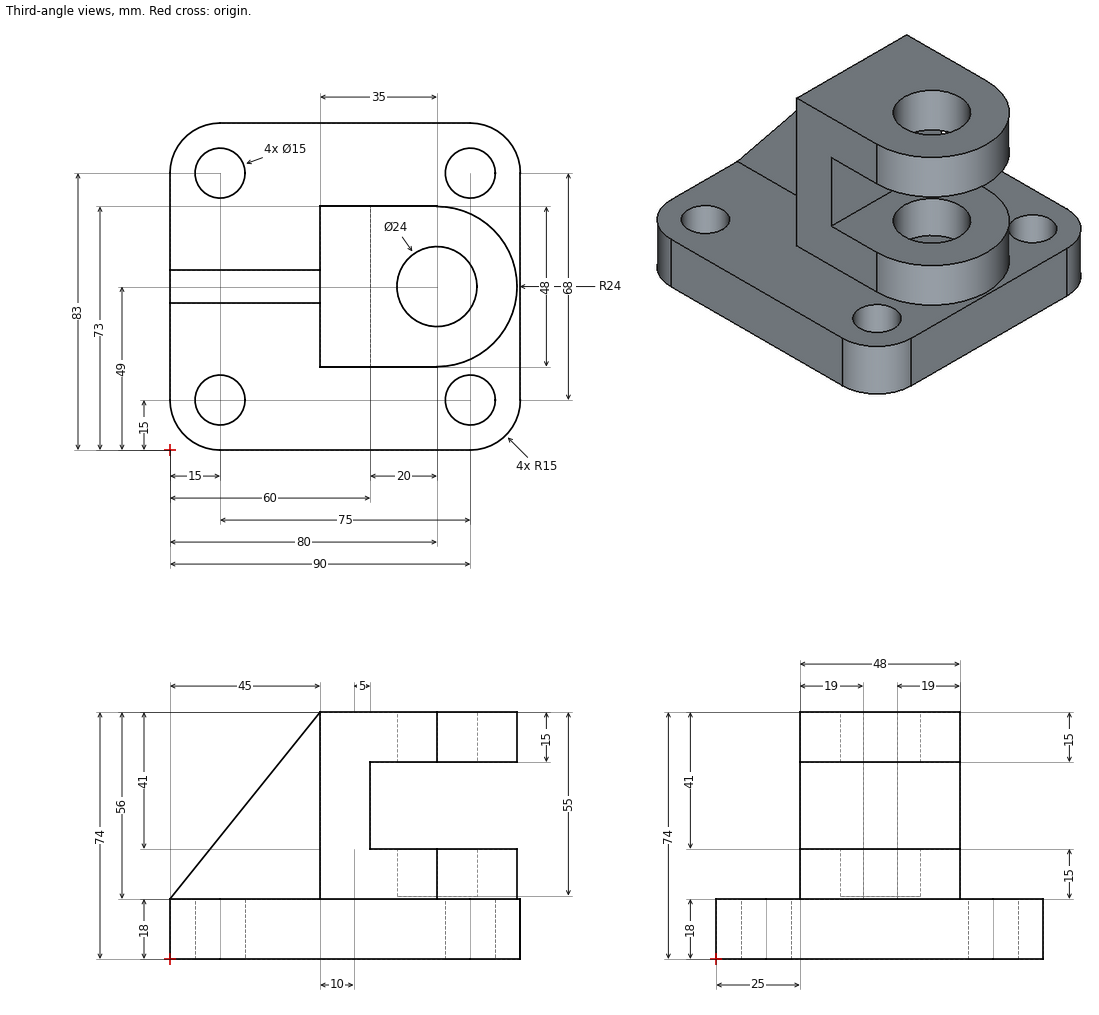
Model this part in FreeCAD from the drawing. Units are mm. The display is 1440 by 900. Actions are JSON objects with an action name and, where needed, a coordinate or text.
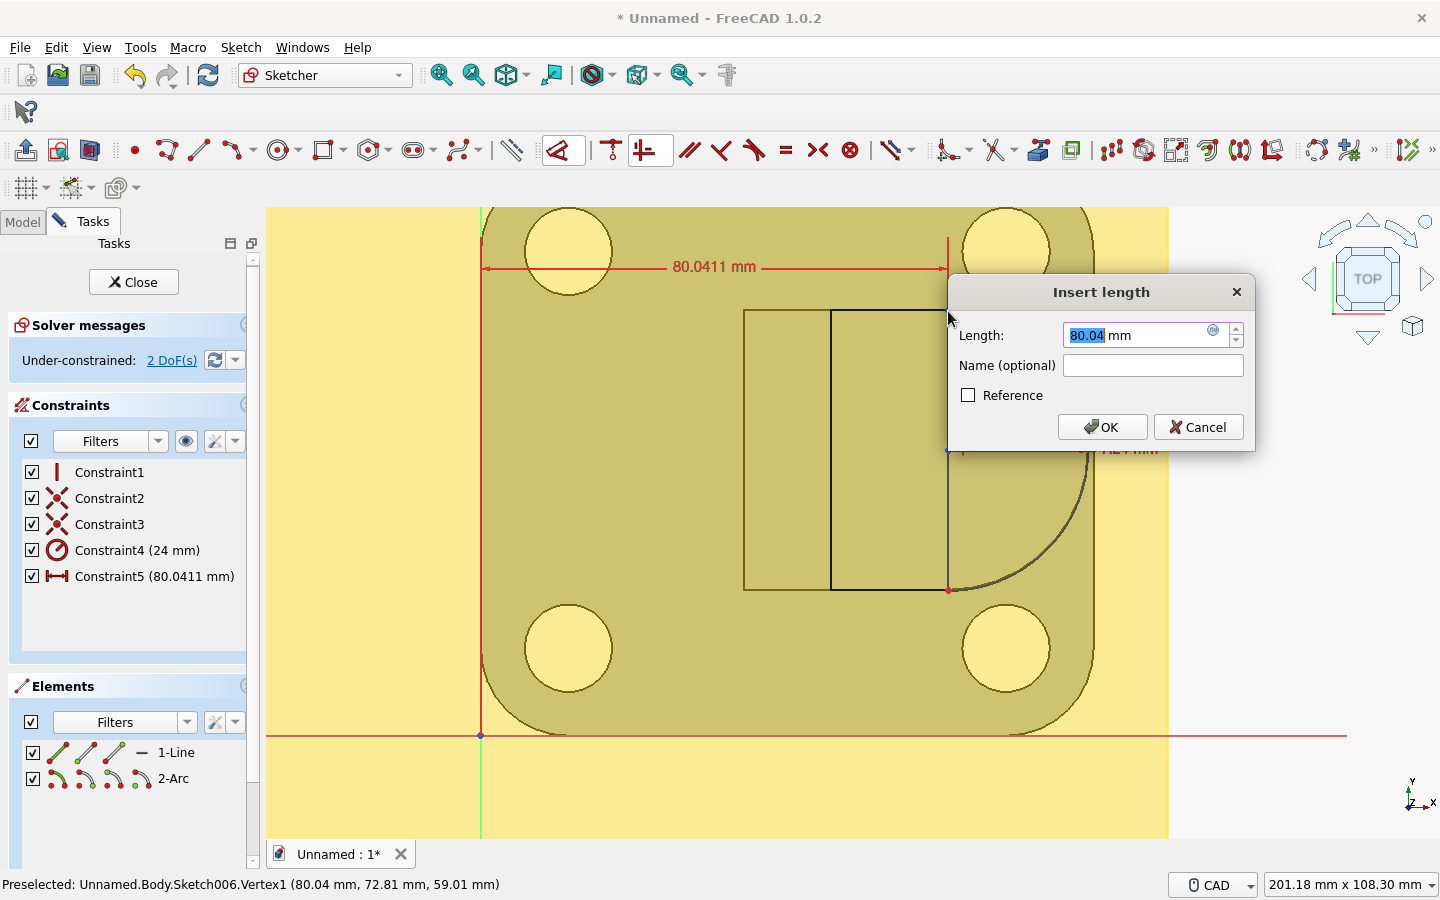
{"action": "type", "text": "80"}
{"action": "key", "text": "Return"}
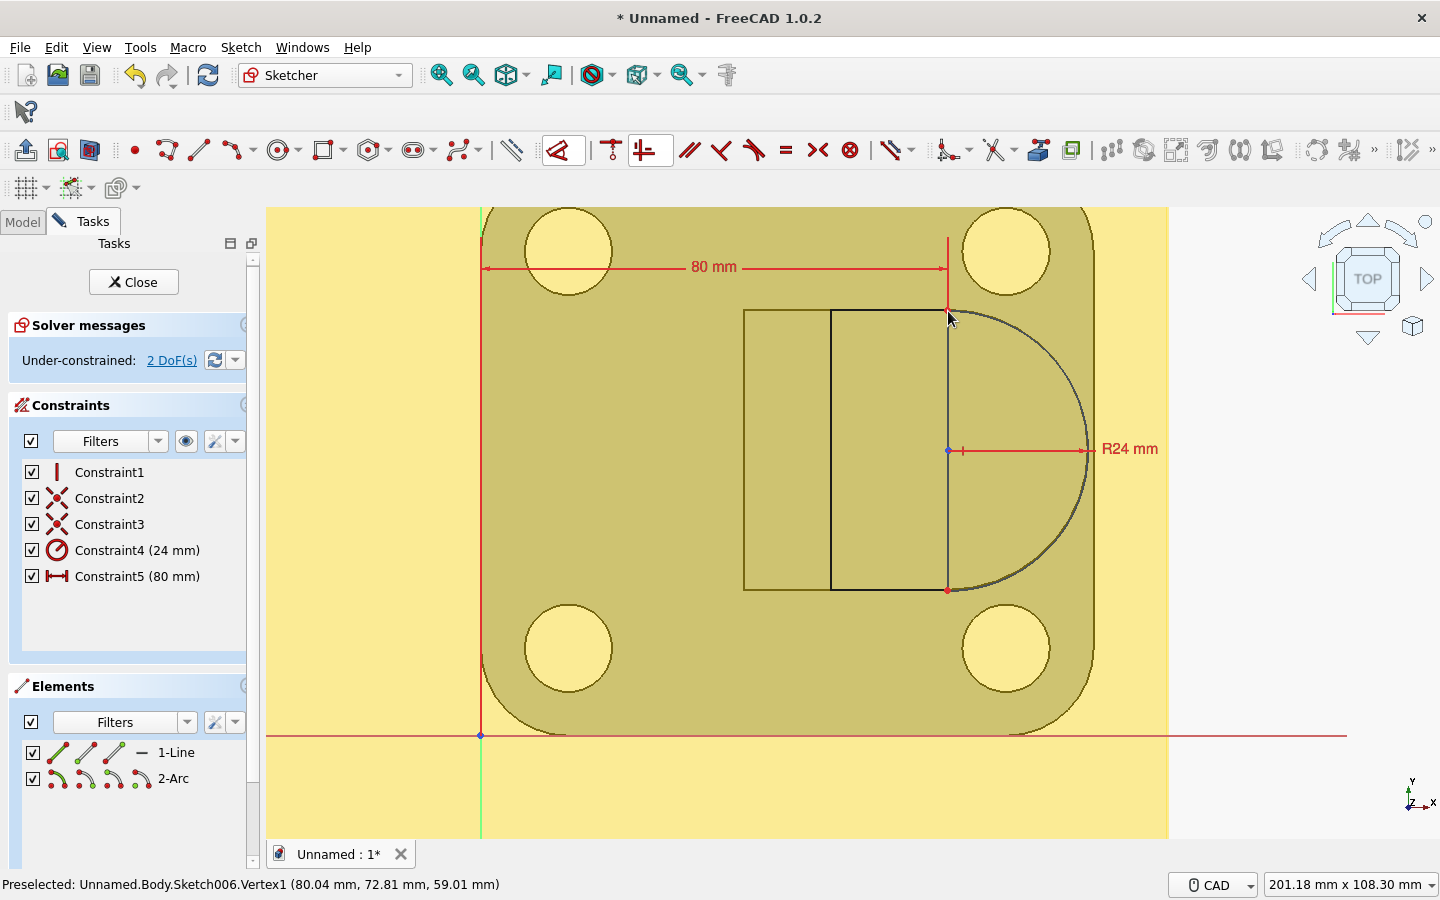
{"action": "left_click", "coordinate": [948, 311]}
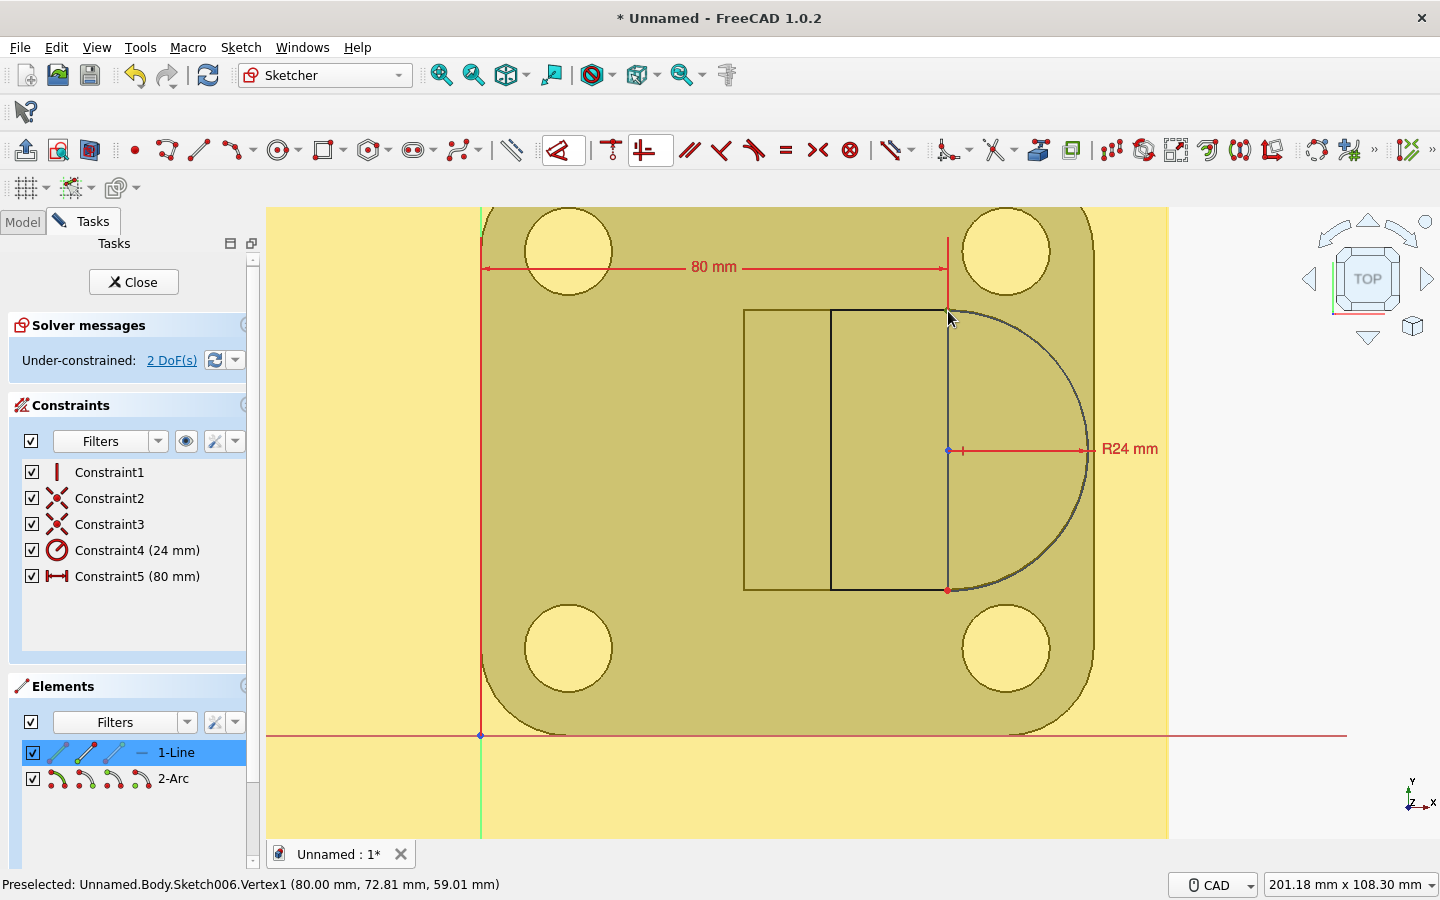
{"action": "left_click", "coordinate": [580, 150]}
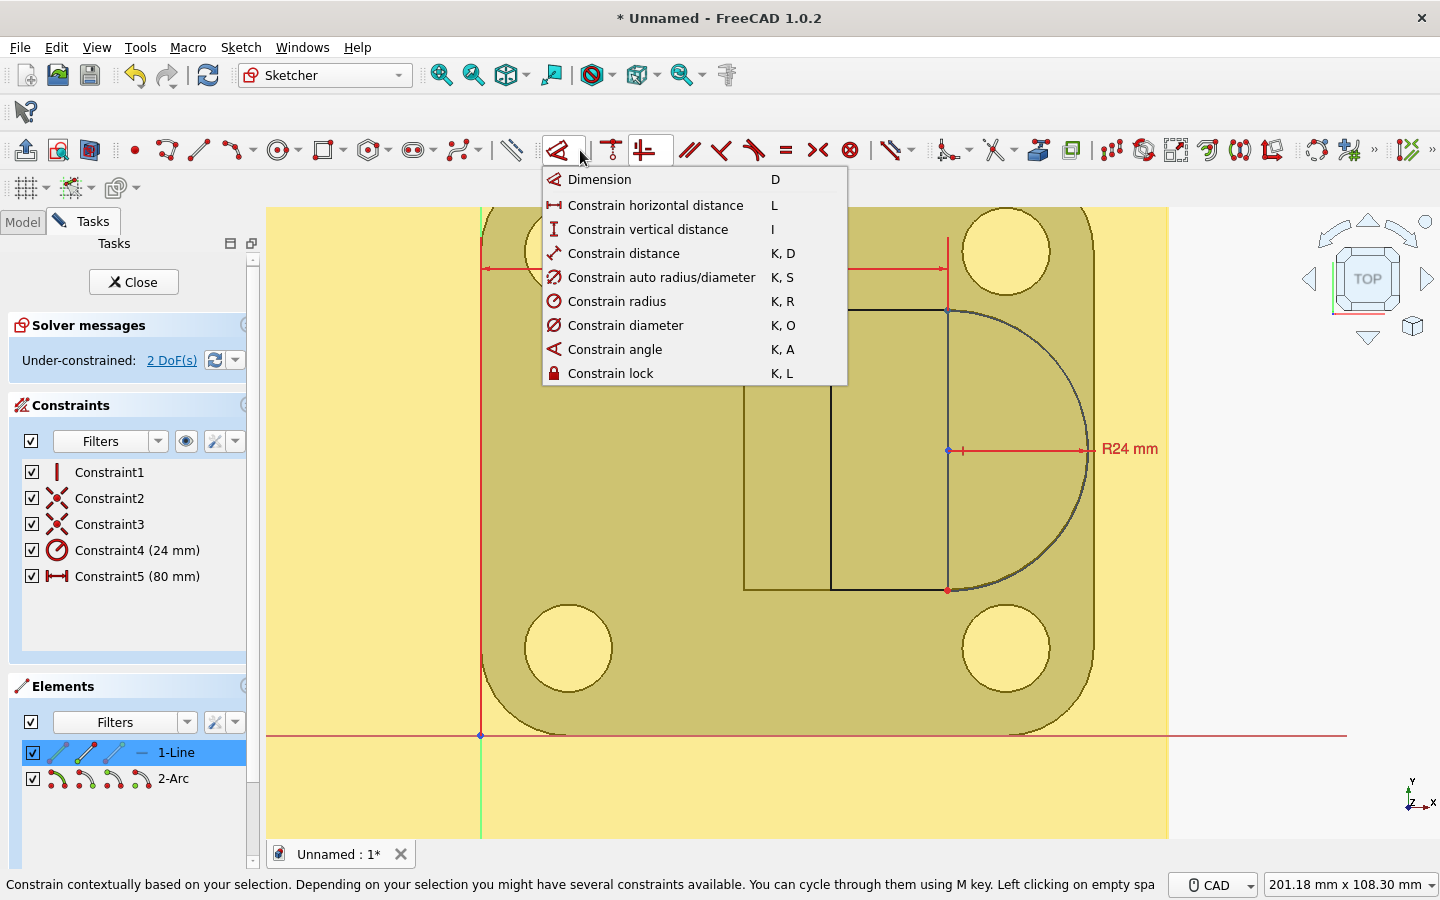
{"action": "left_click", "coordinate": [695, 229]}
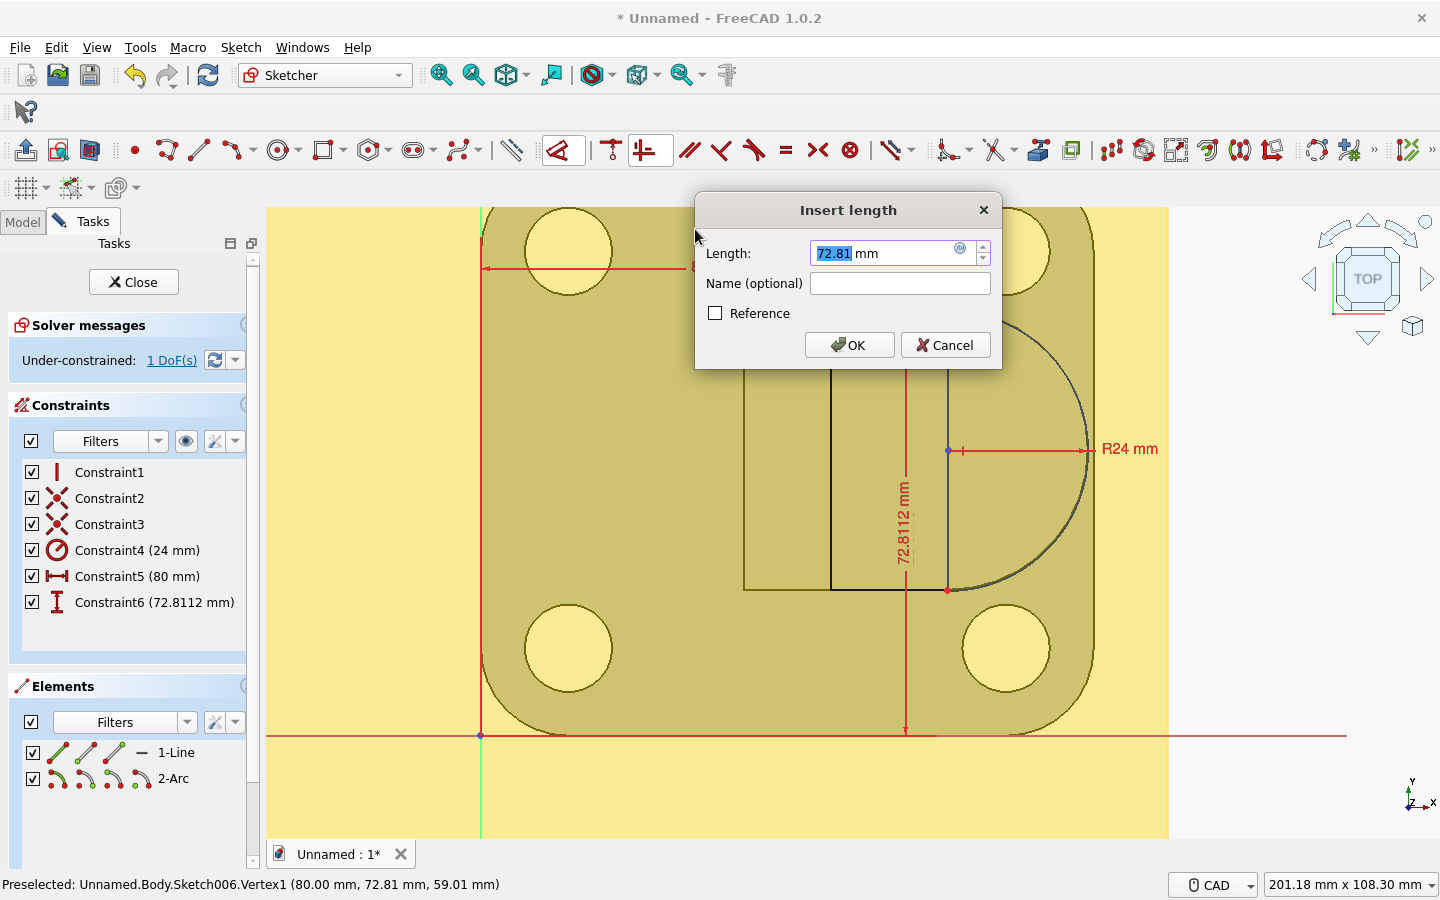
{"action": "type", "text": "73"}
{"action": "key", "text": "Return"}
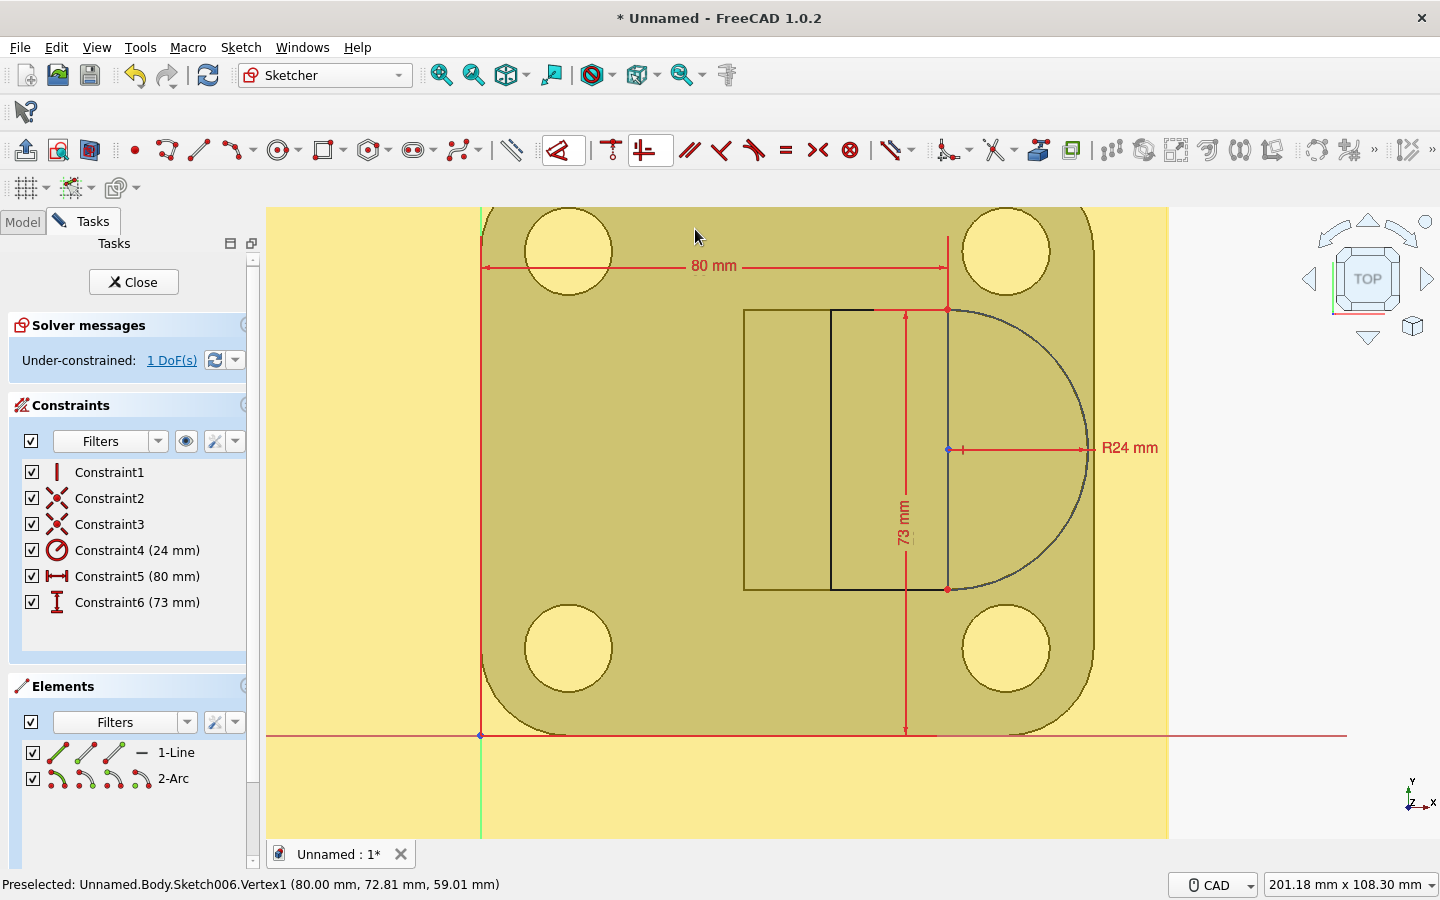
{"action": "left_click", "coordinate": [948, 450]}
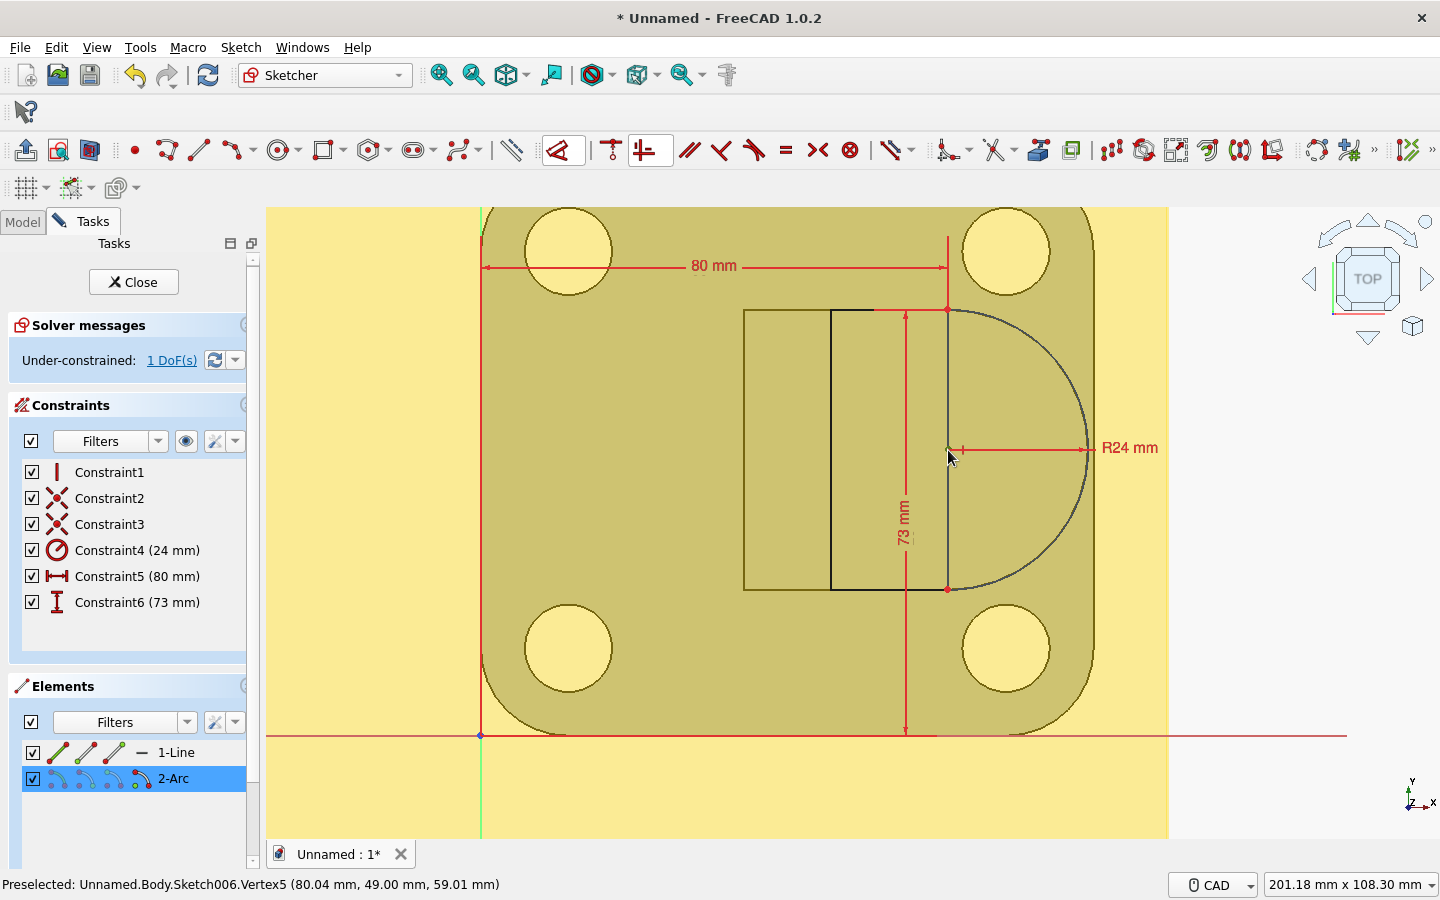
{"action": "left_click", "coordinate": [580, 150]}